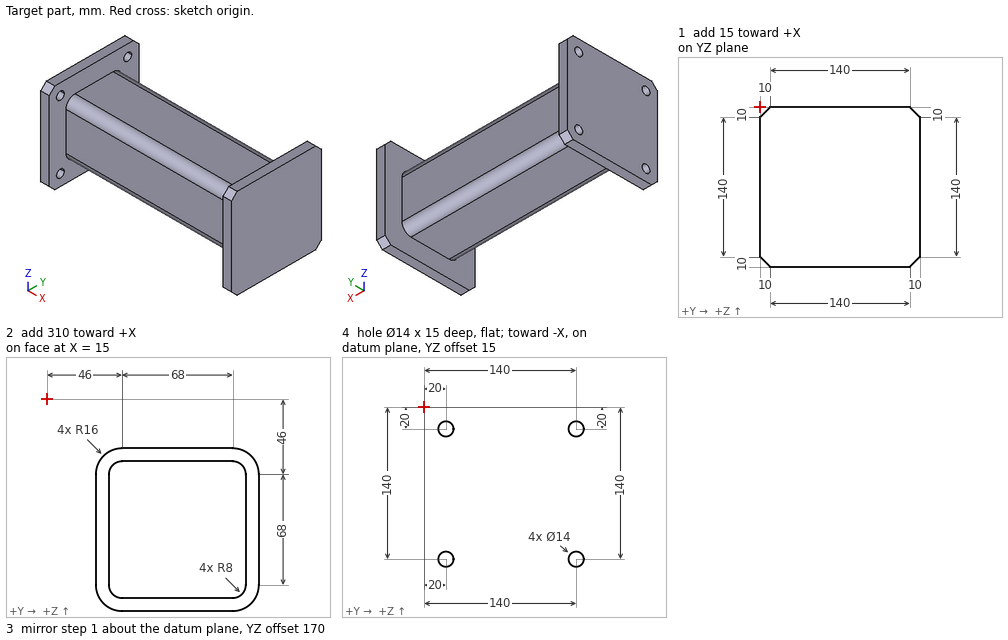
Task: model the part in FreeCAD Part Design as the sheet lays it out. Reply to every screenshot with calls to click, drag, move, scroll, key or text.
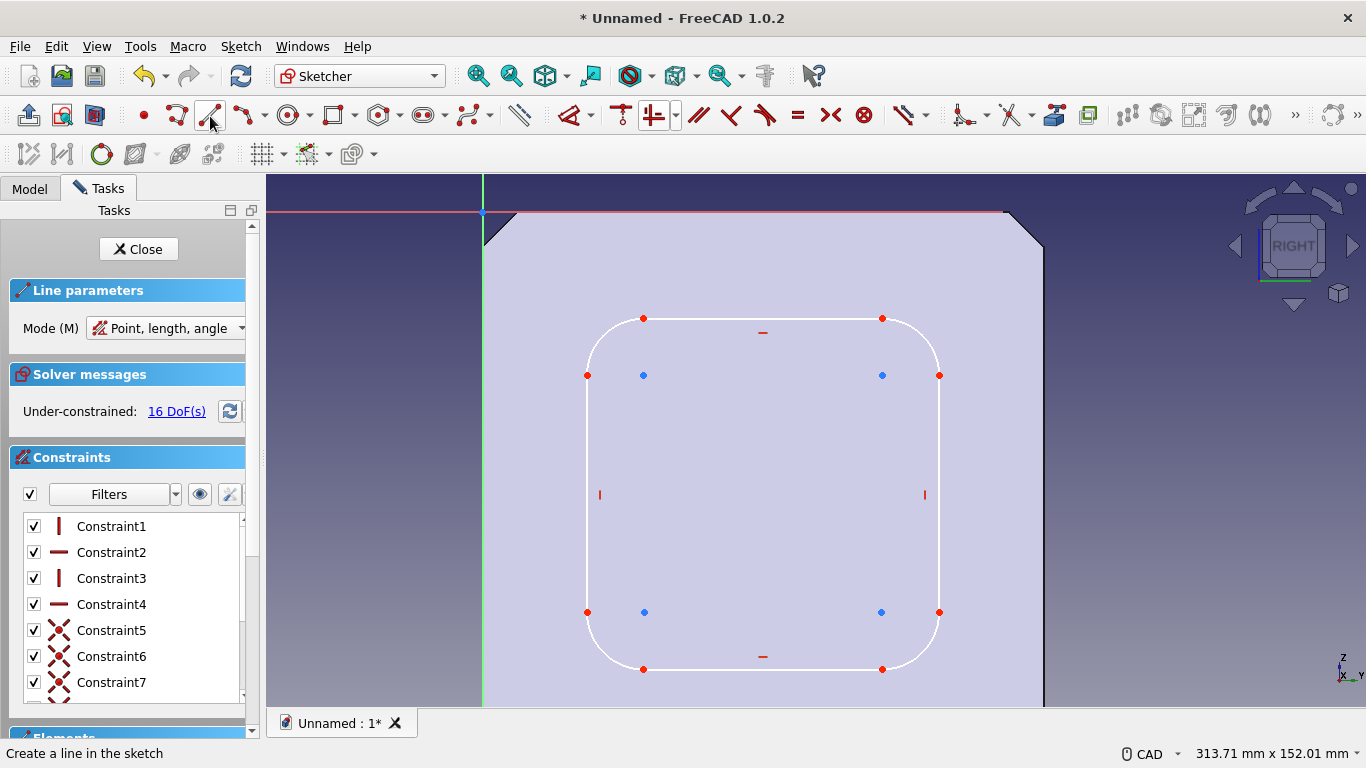
click(910, 374)
click(910, 612)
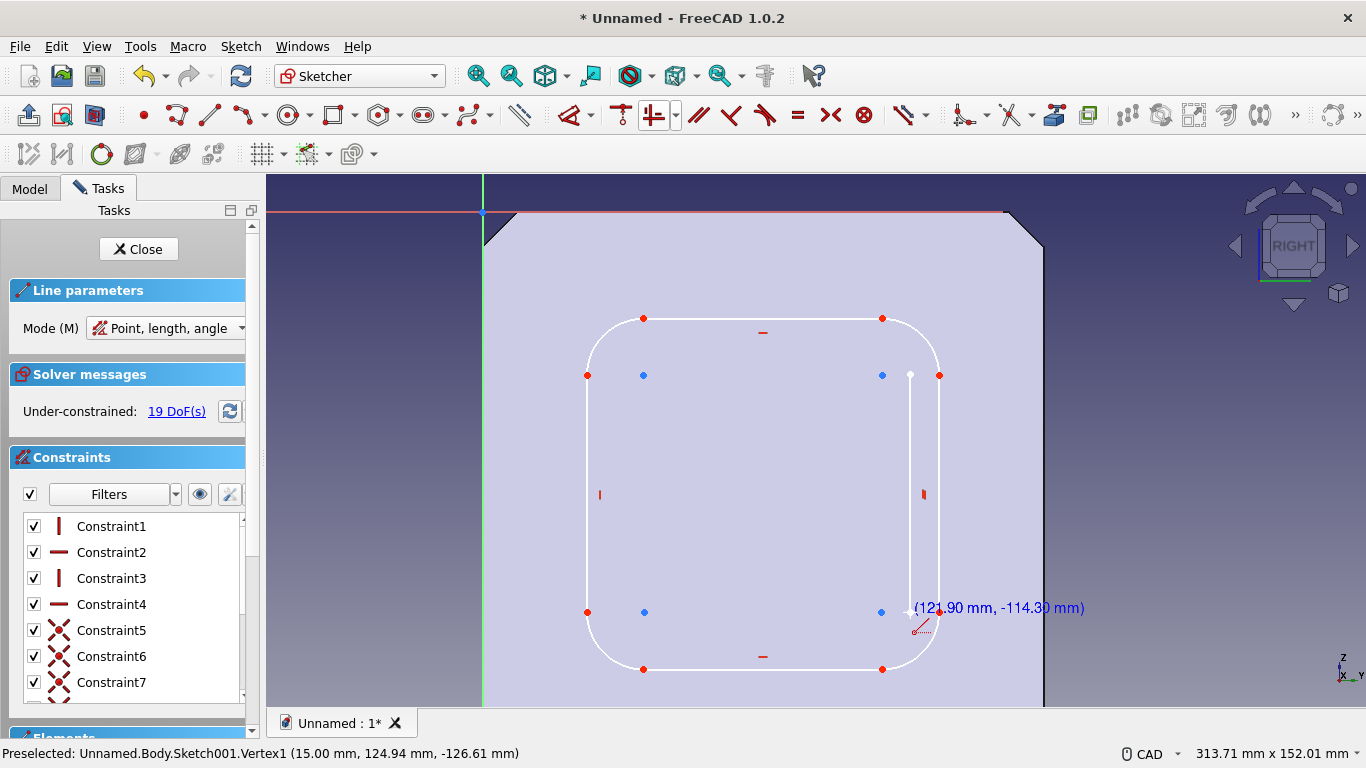
click(882, 640)
click(644, 640)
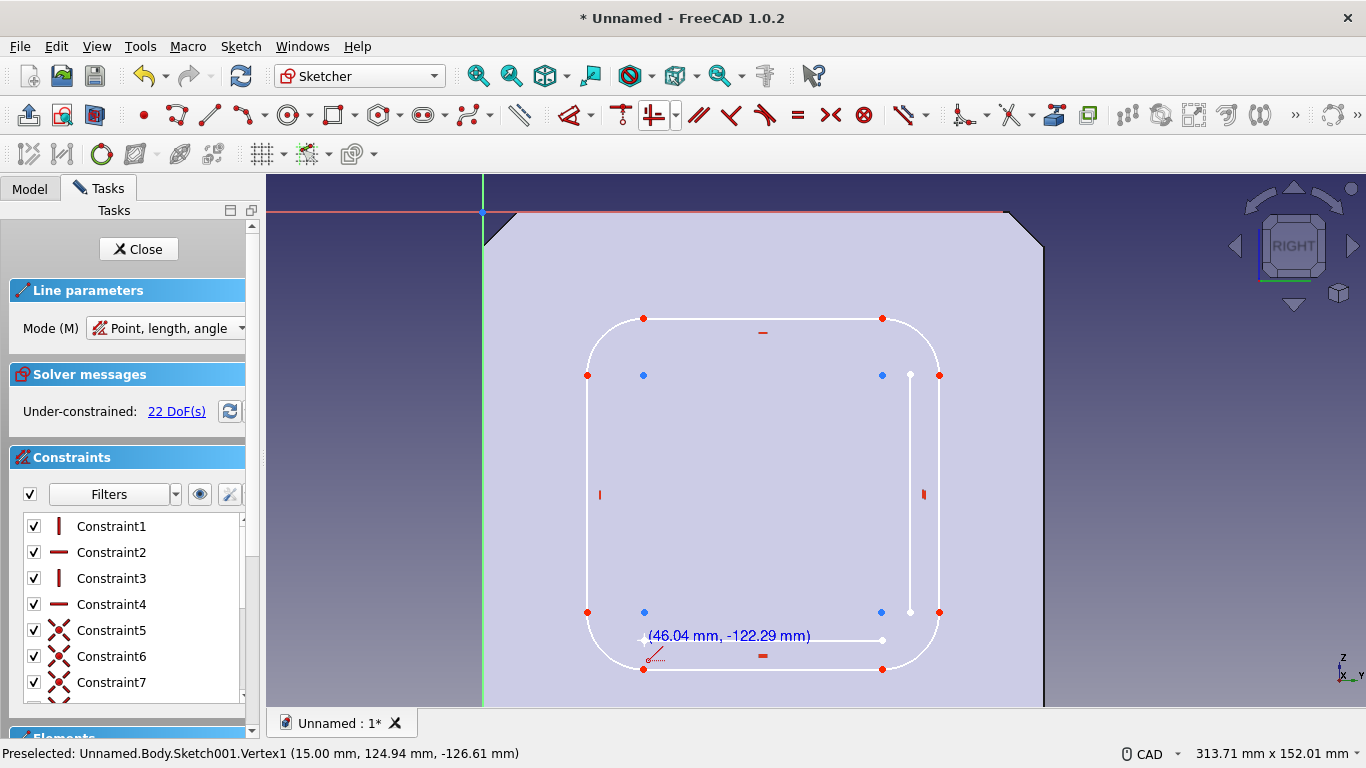
click(616, 612)
click(616, 374)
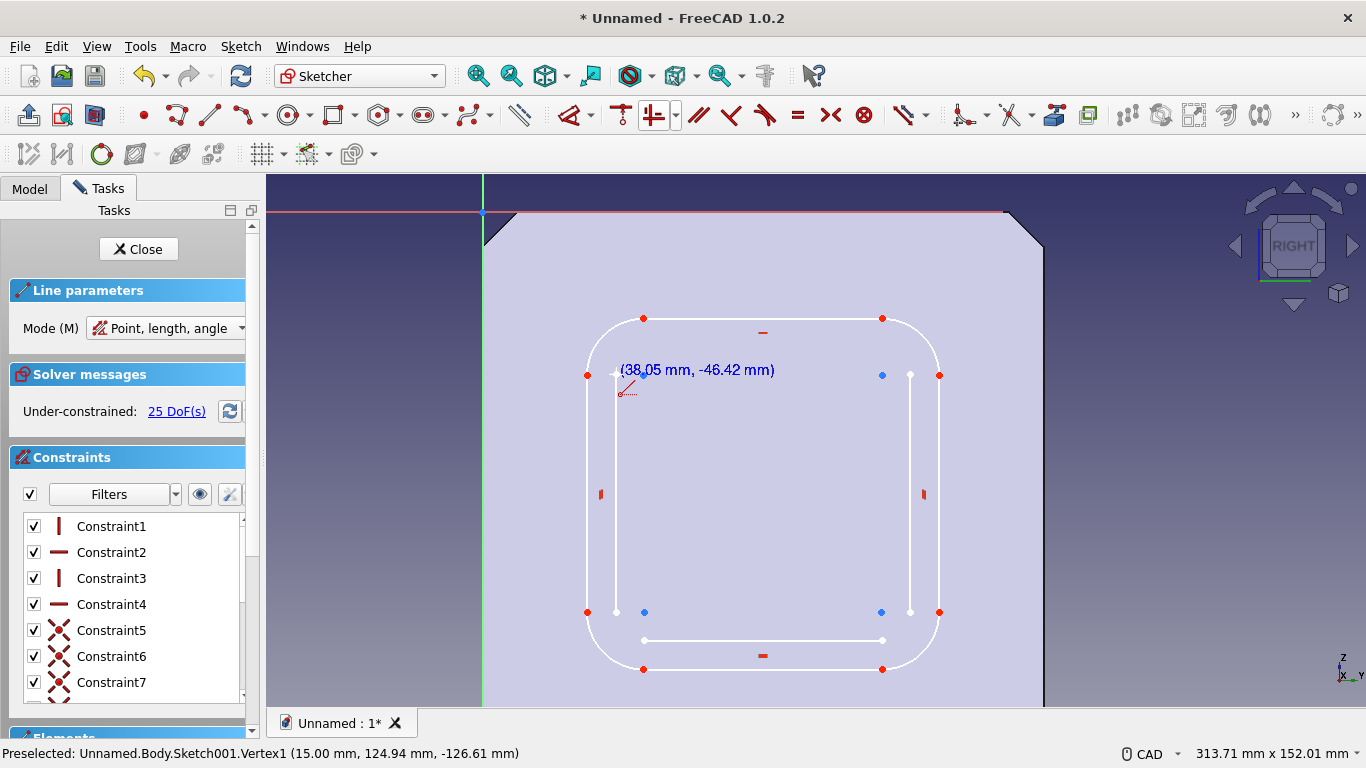
click(644, 345)
click(882, 345)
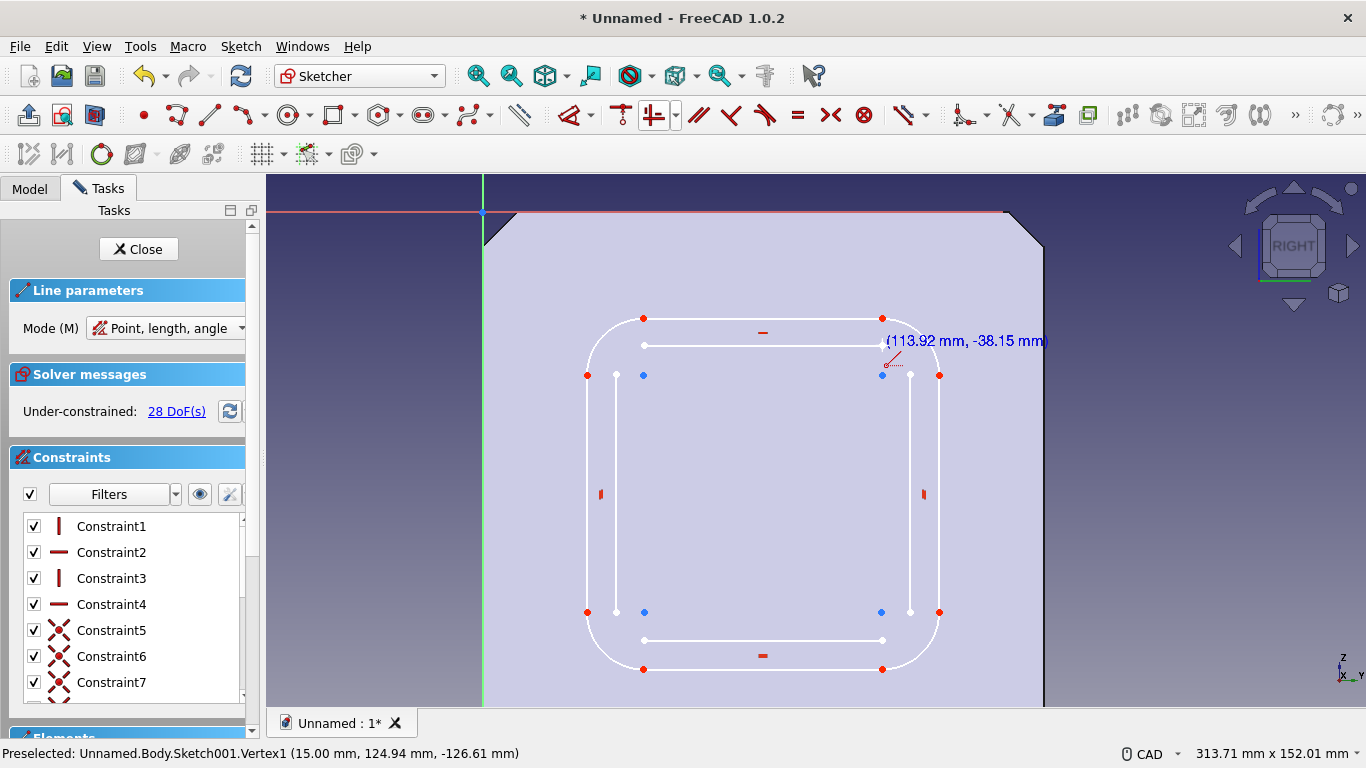
key(g)
key(3)
key(a)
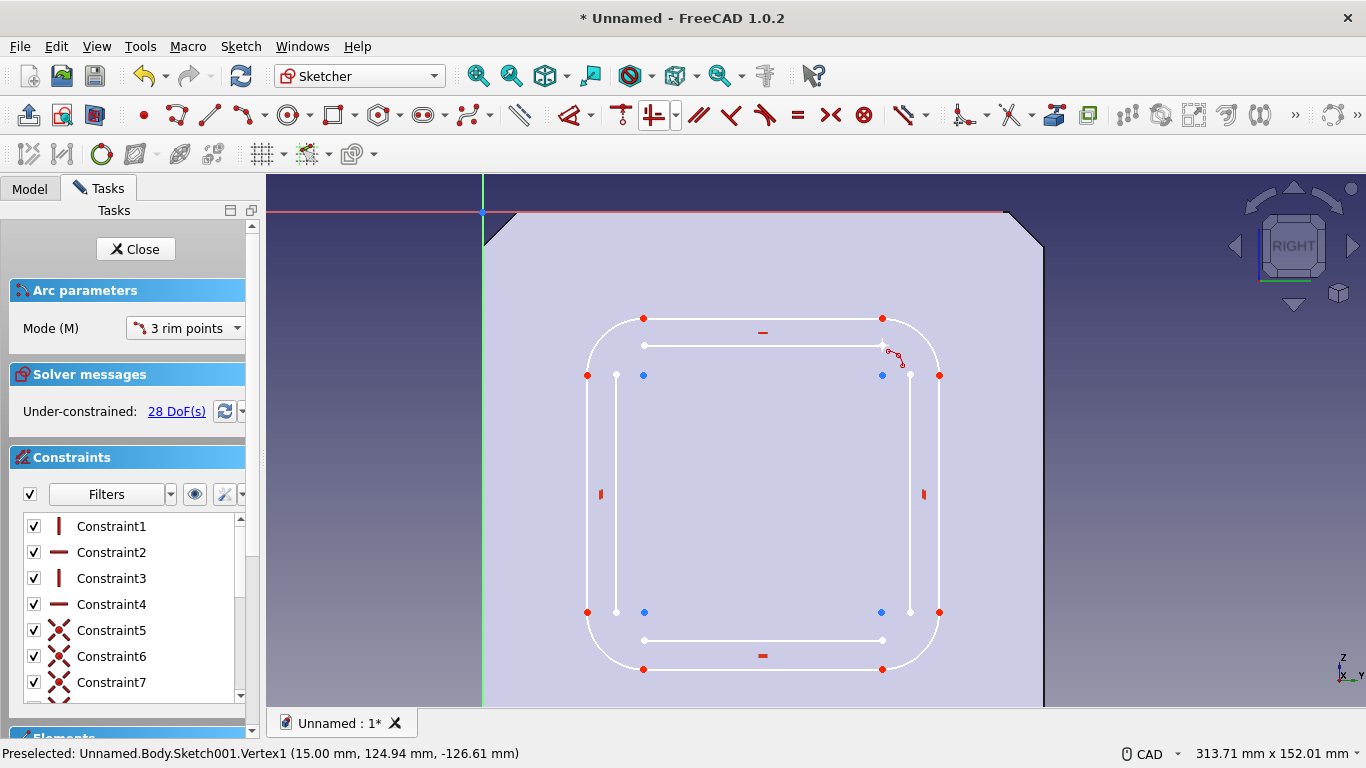
click(910, 613)
click(882, 641)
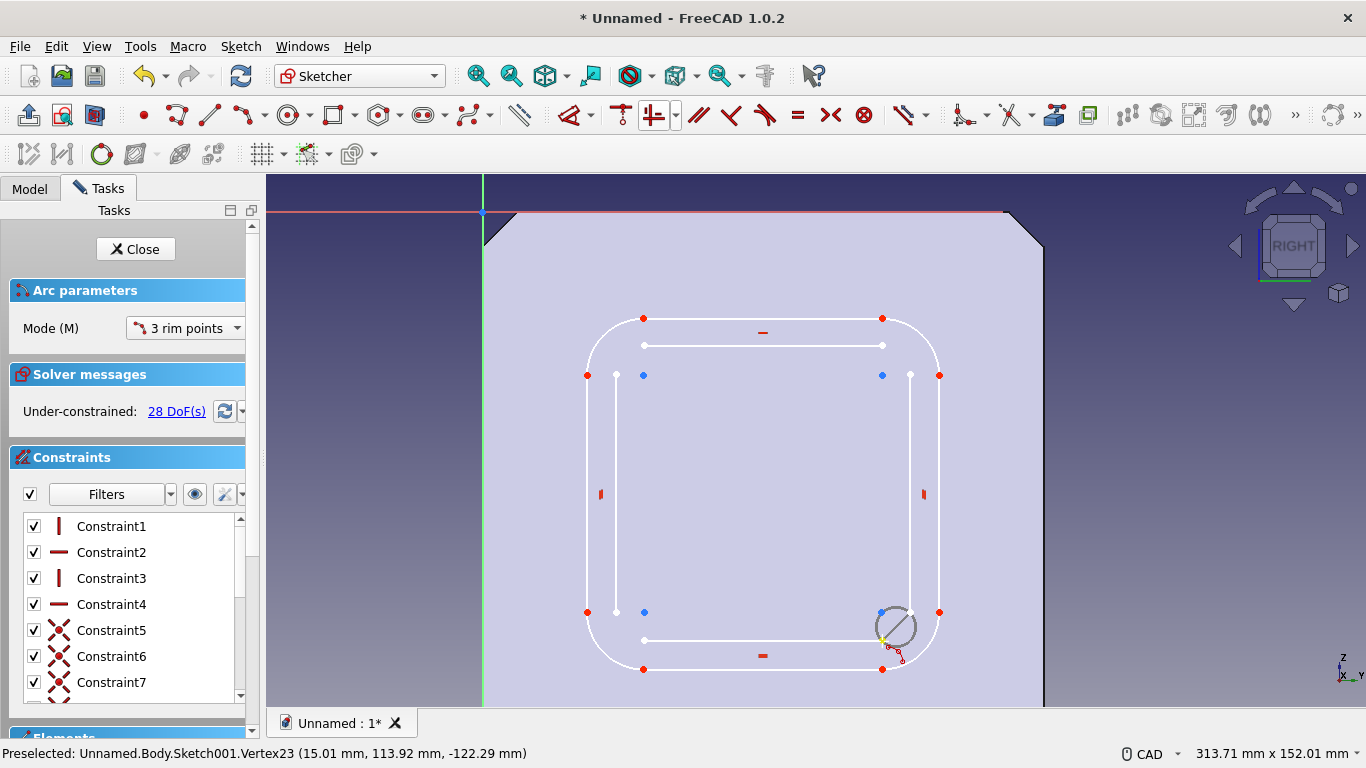
scroll(902, 632, up, 4)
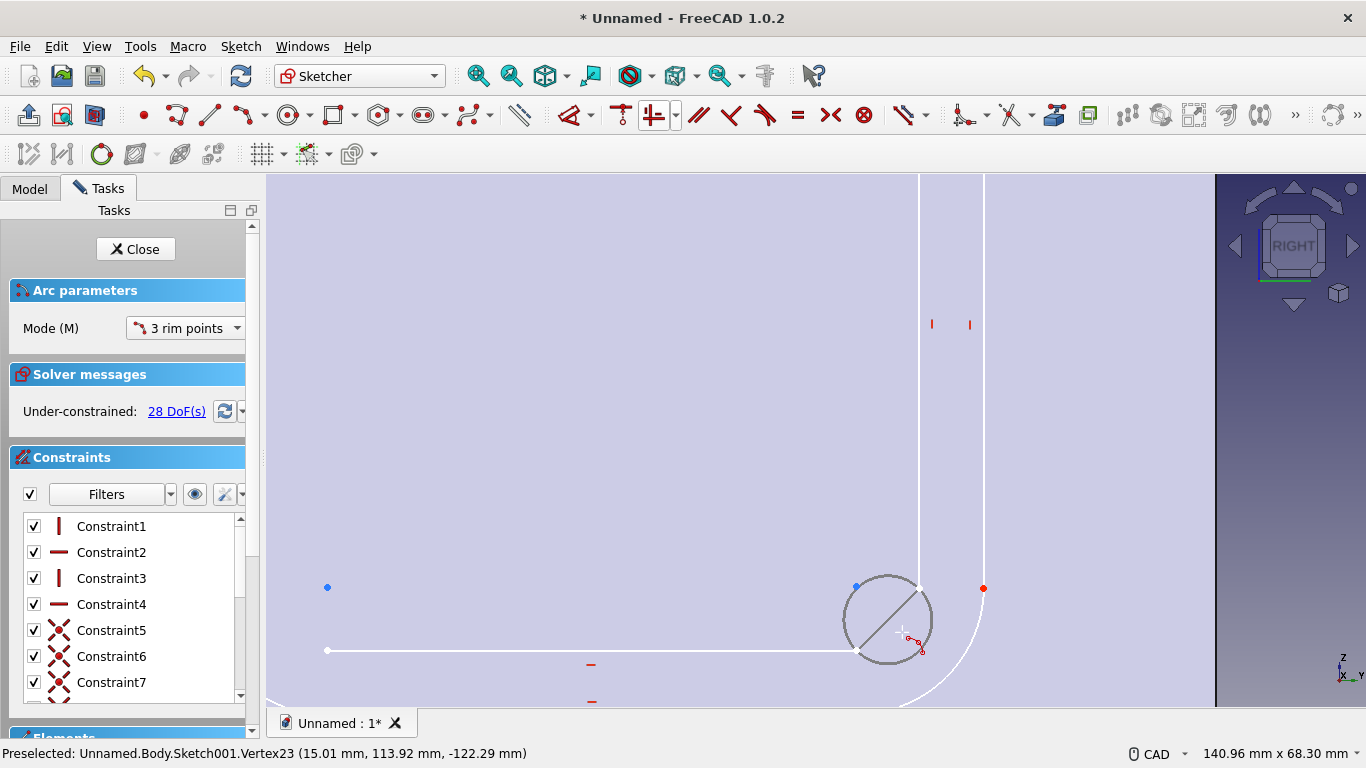
click(902, 630)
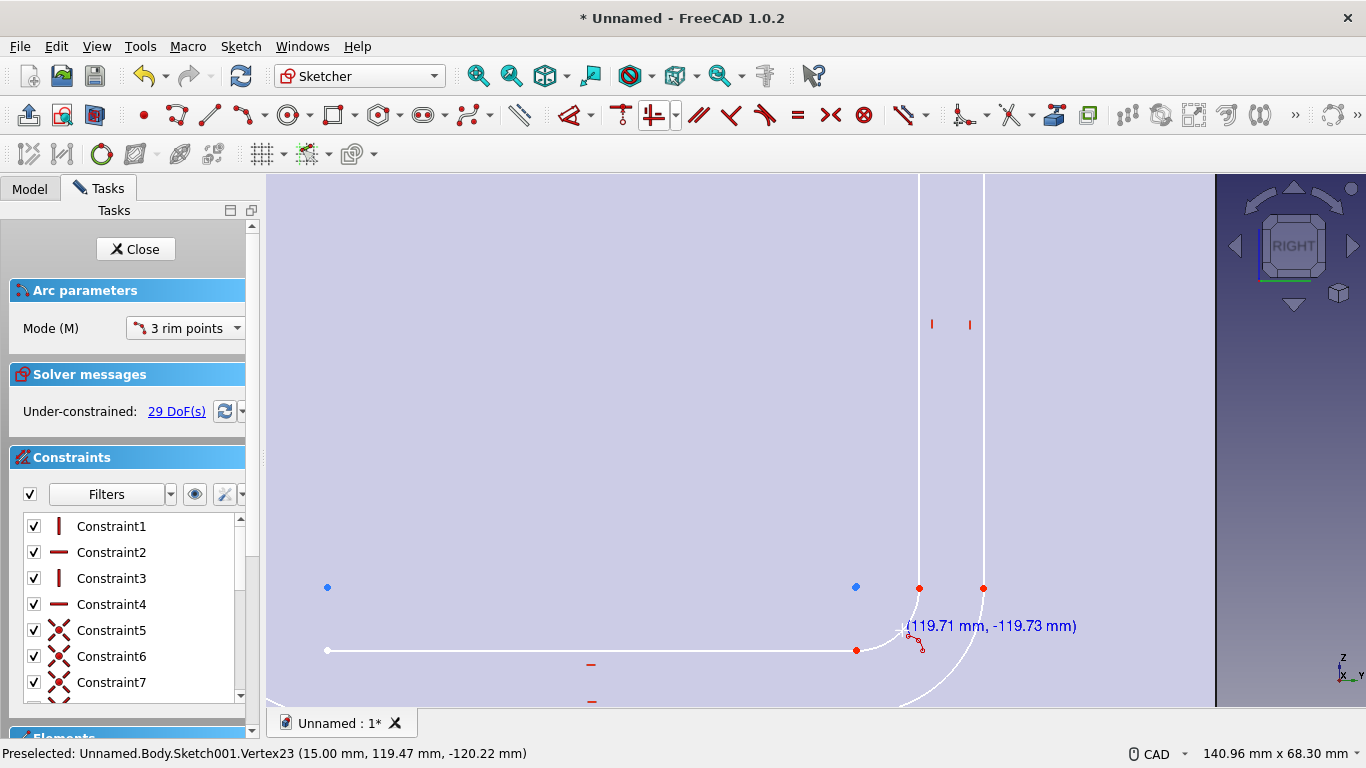
click(327, 651)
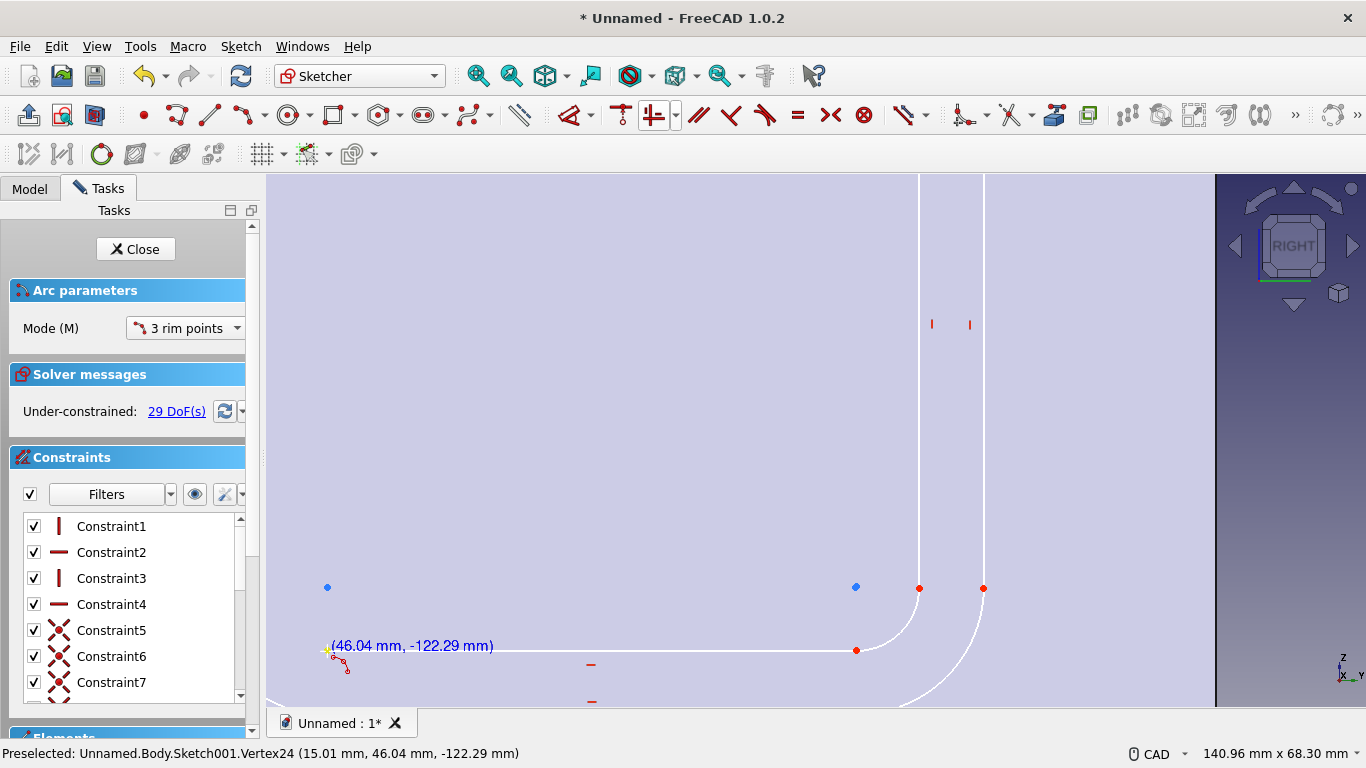
scroll(865, 542, down, 6)